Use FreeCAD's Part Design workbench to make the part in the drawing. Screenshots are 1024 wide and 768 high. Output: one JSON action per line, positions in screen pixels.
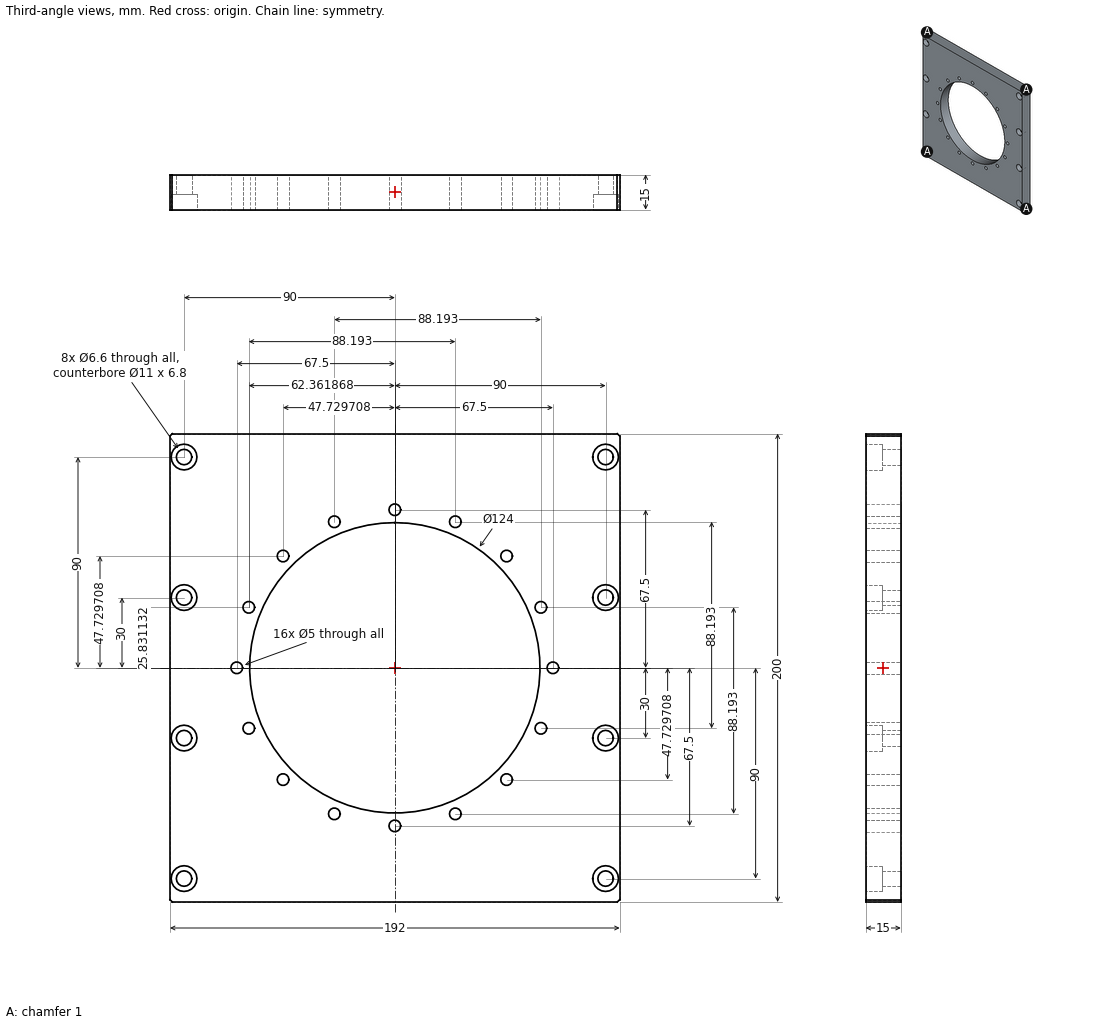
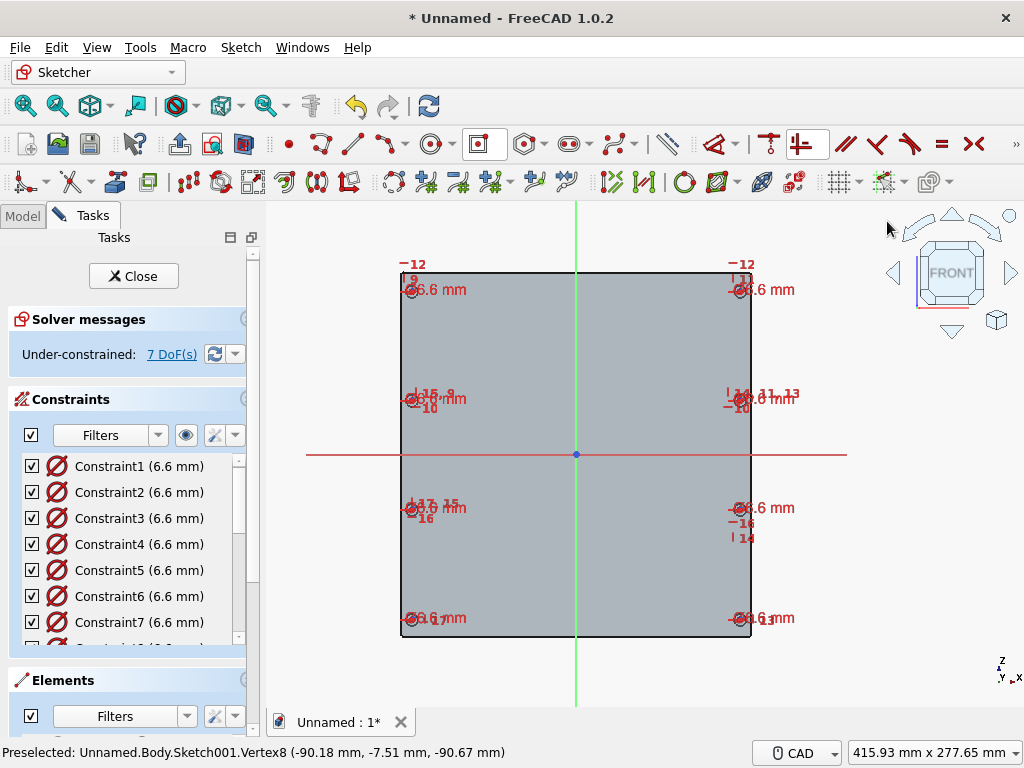
{"action": "left_click", "coordinate": [740, 620]}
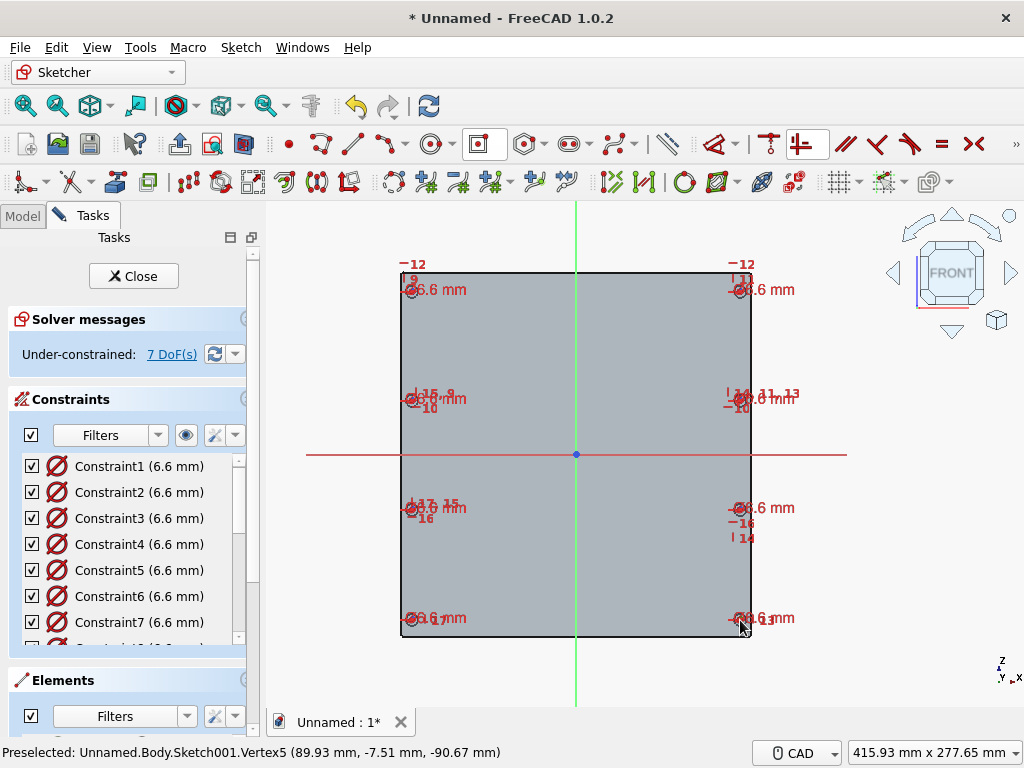
{"action": "left_click", "coordinate": [412, 620]}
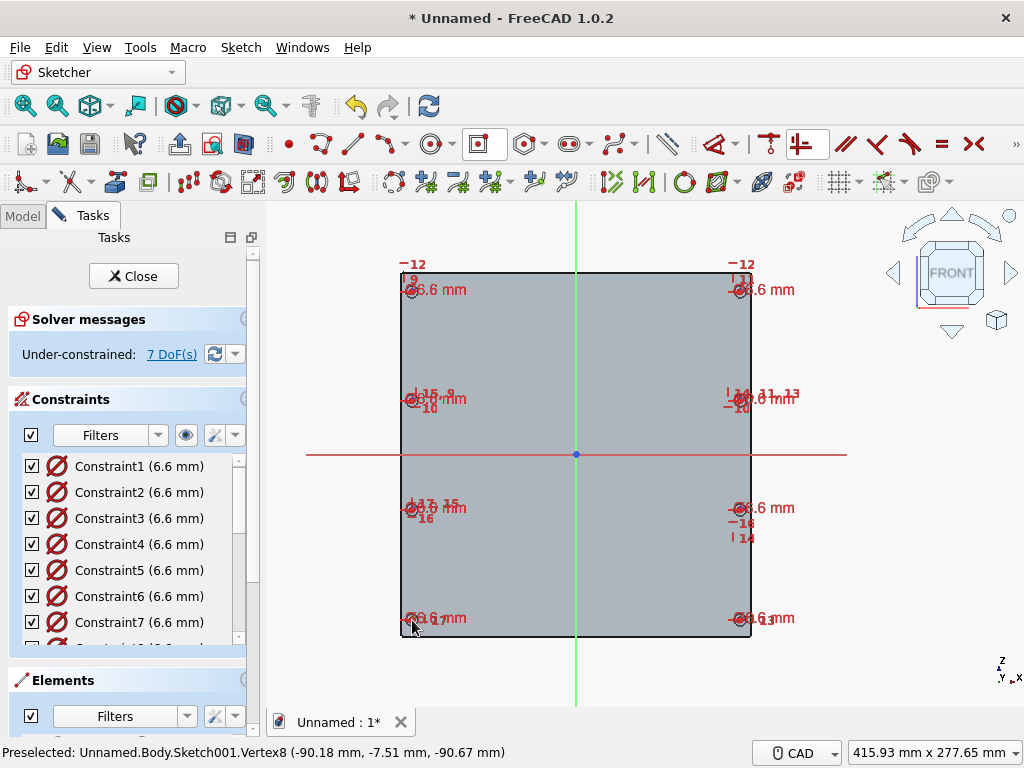
{"action": "key", "text": "h"}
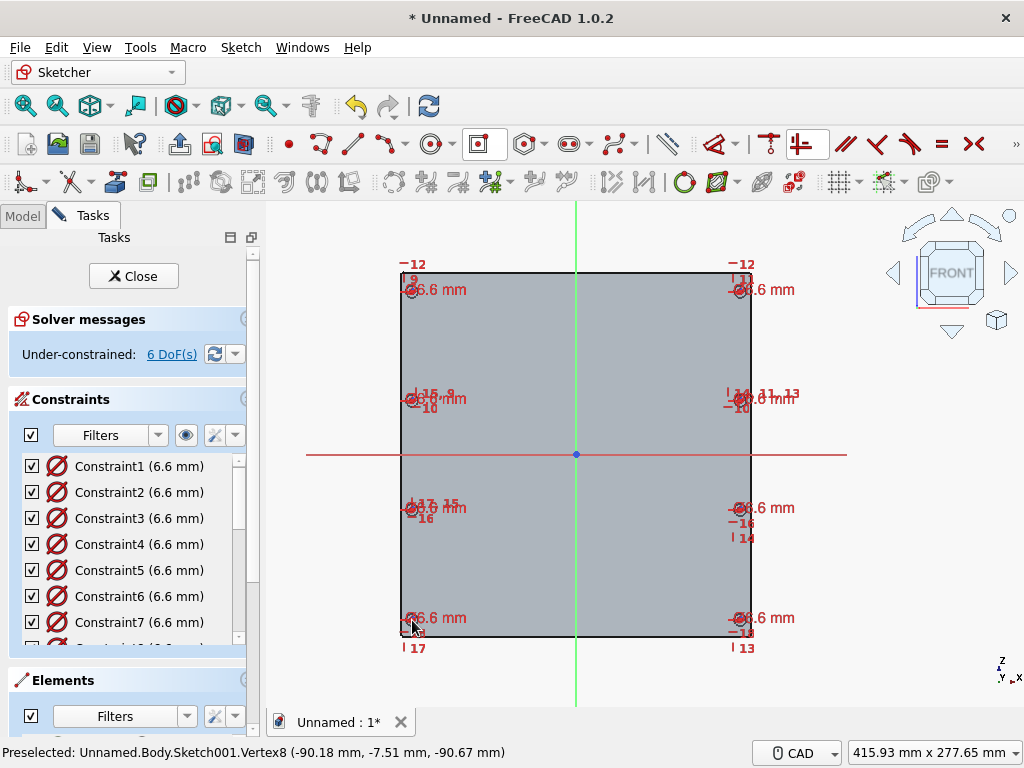
{"action": "left_click", "coordinate": [714, 144]}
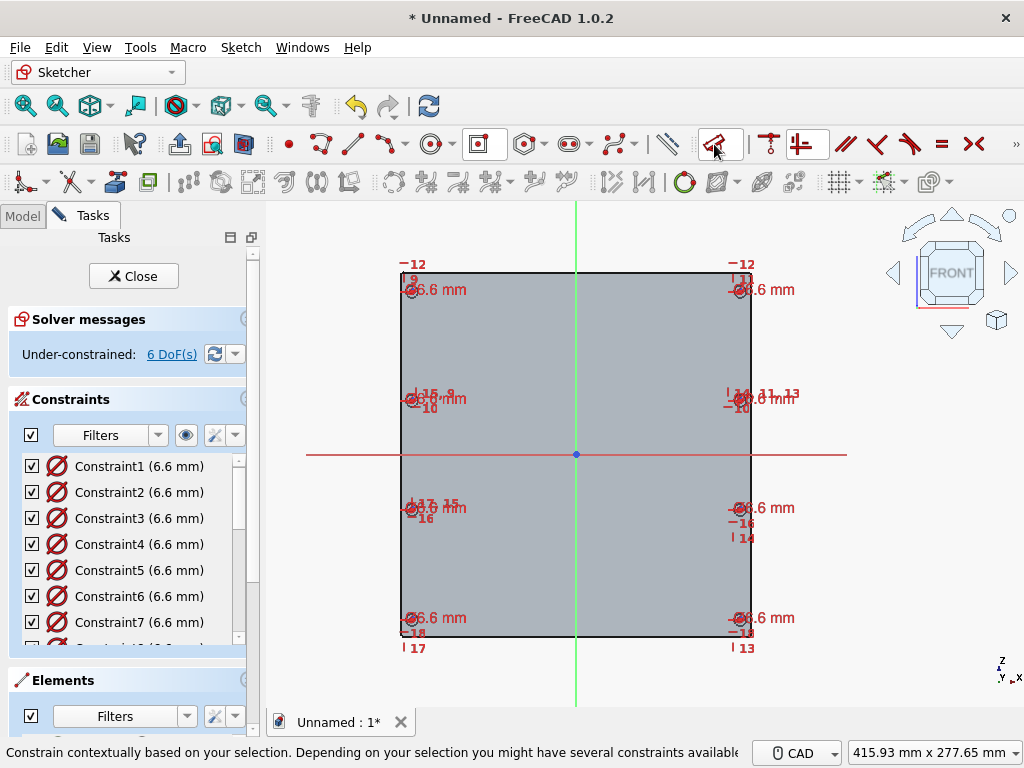
{"action": "left_click", "coordinate": [412, 292]}
{"action": "left_click", "coordinate": [494, 258]}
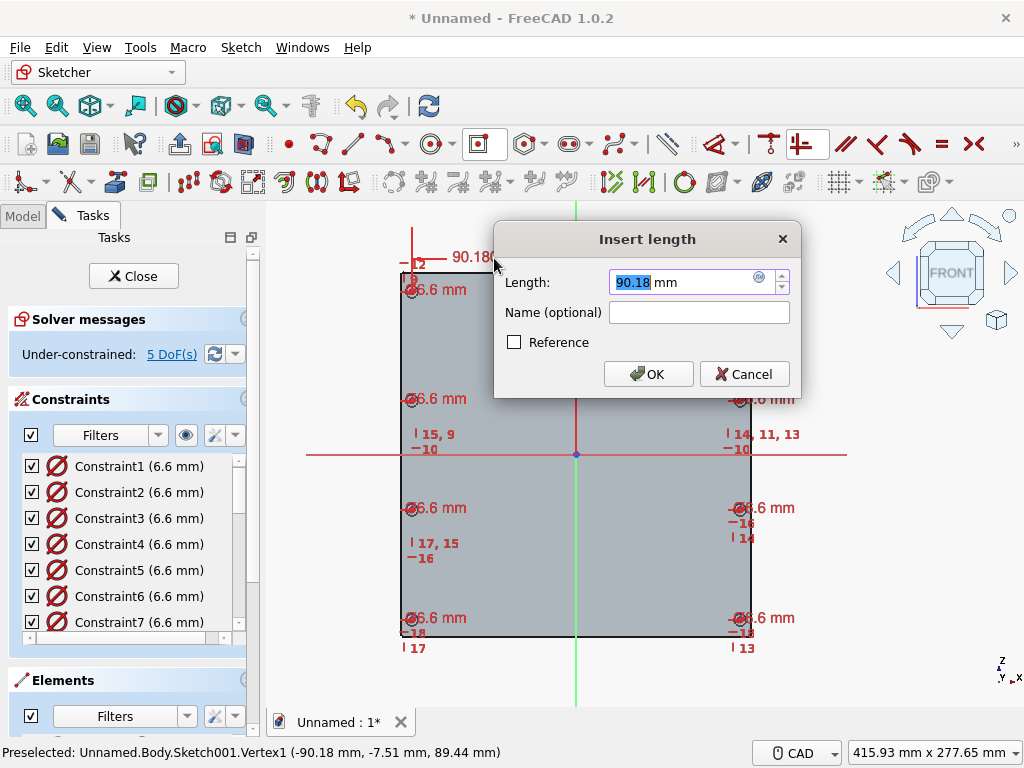
{"action": "type", "text": "90"}
{"action": "key", "text": "Return"}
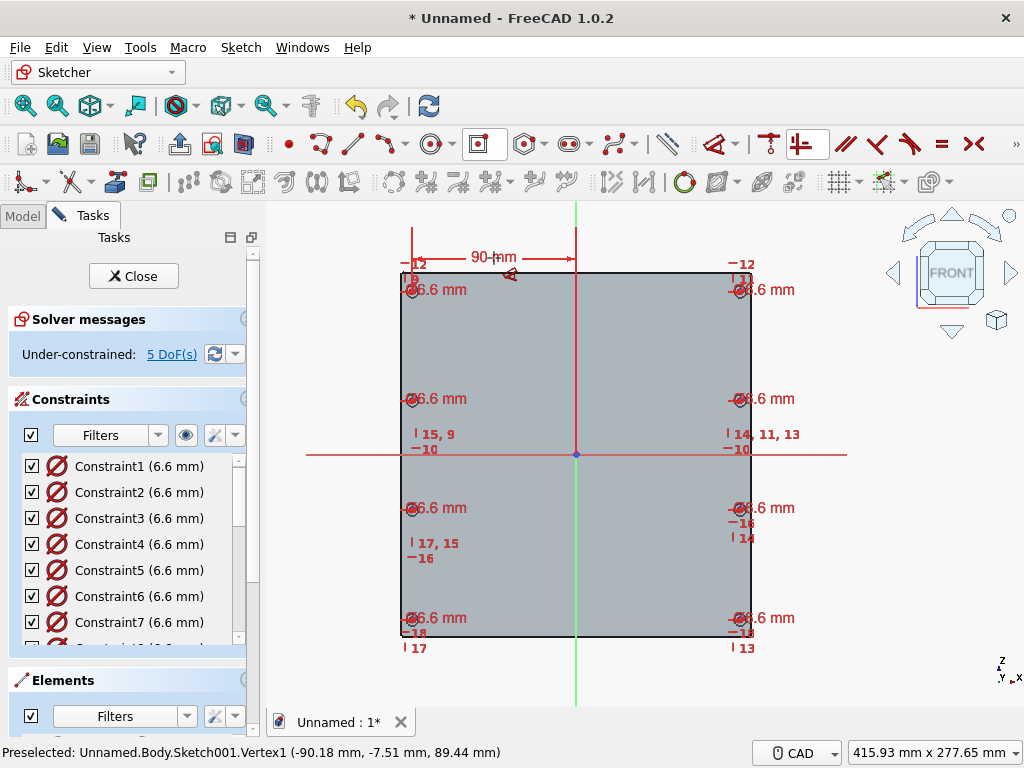
{"action": "left_click", "coordinate": [412, 292]}
{"action": "left_click", "coordinate": [378, 373]}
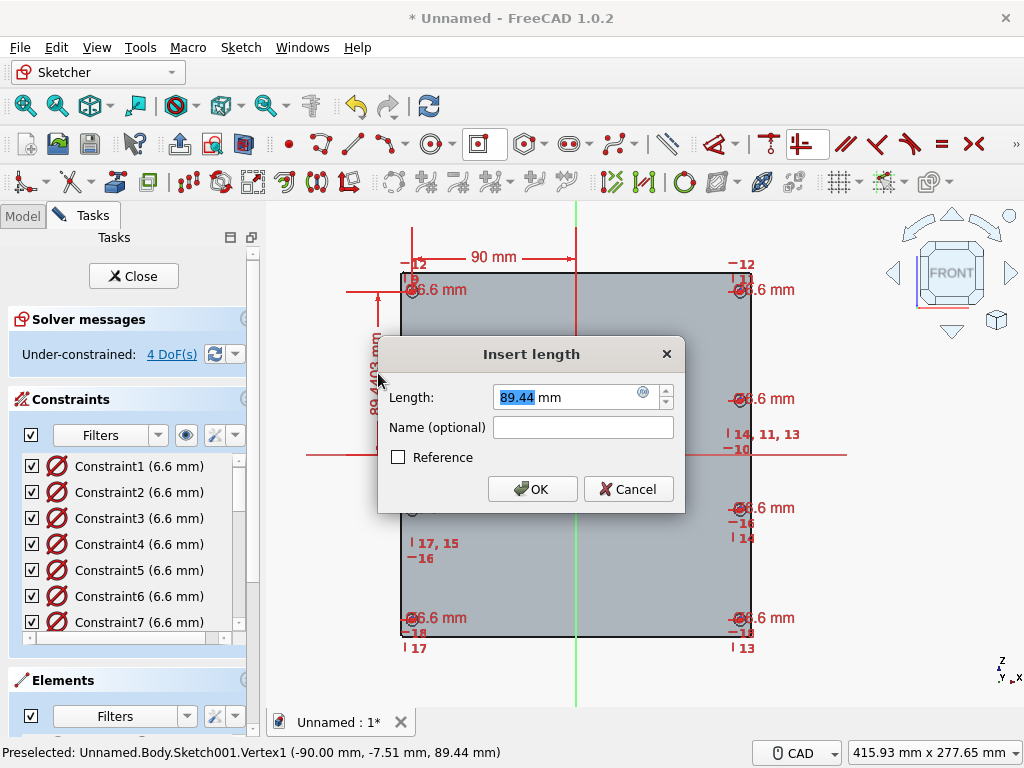
{"action": "type", "text": "90"}
{"action": "key", "text": "Return"}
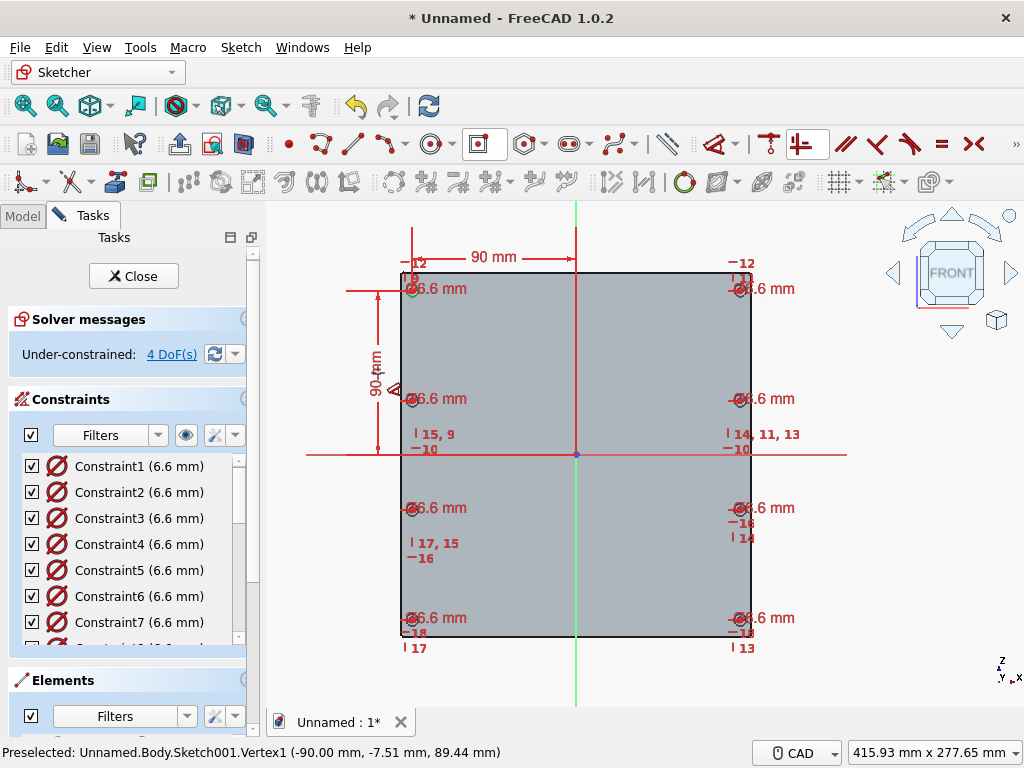
{"action": "left_click", "coordinate": [412, 401]}
{"action": "left_click", "coordinate": [378, 428]}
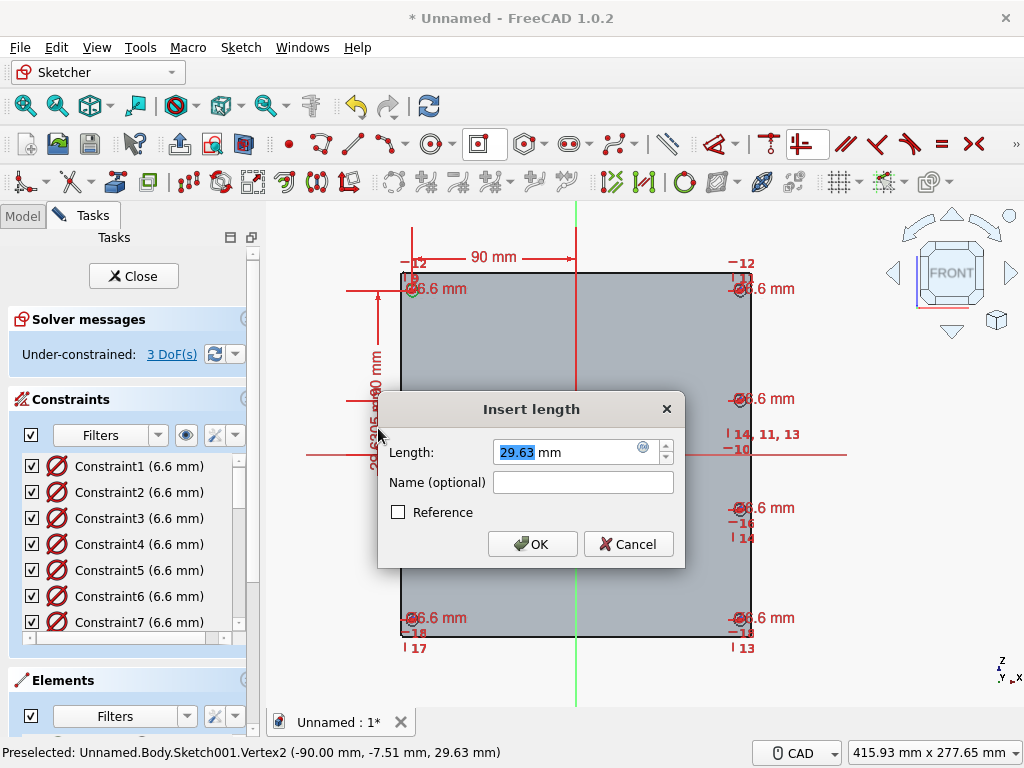
{"action": "type", "text": "30"}
{"action": "key", "text": "Return"}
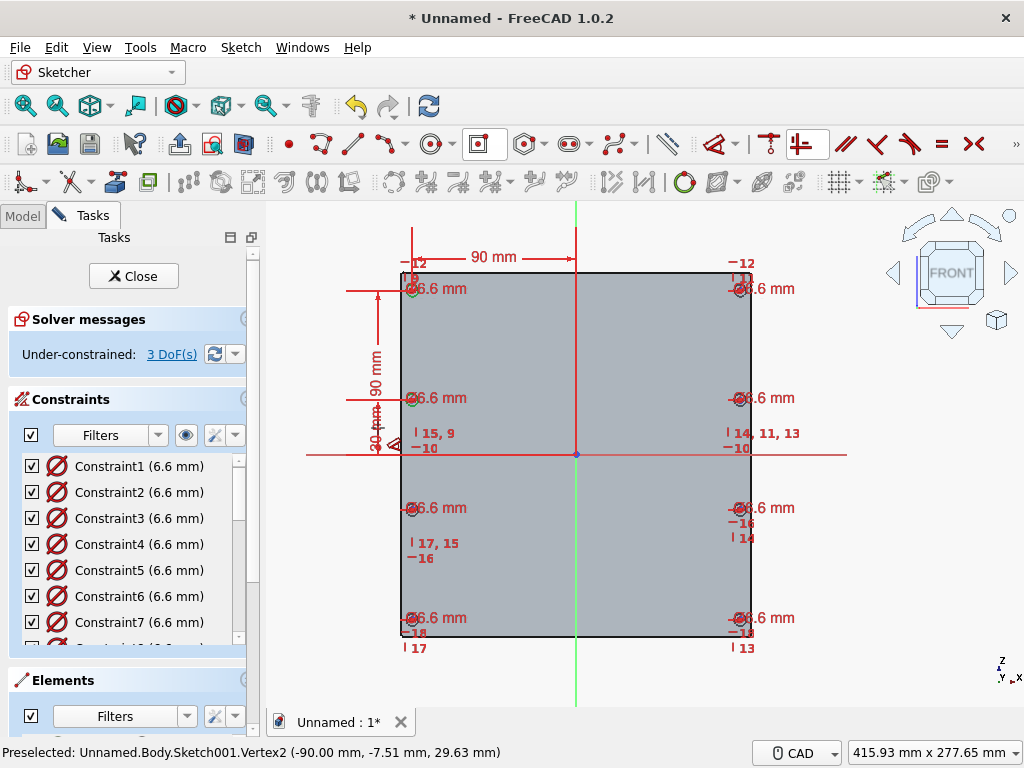
{"action": "left_click", "coordinate": [740, 400]}
{"action": "left_click", "coordinate": [658, 366]}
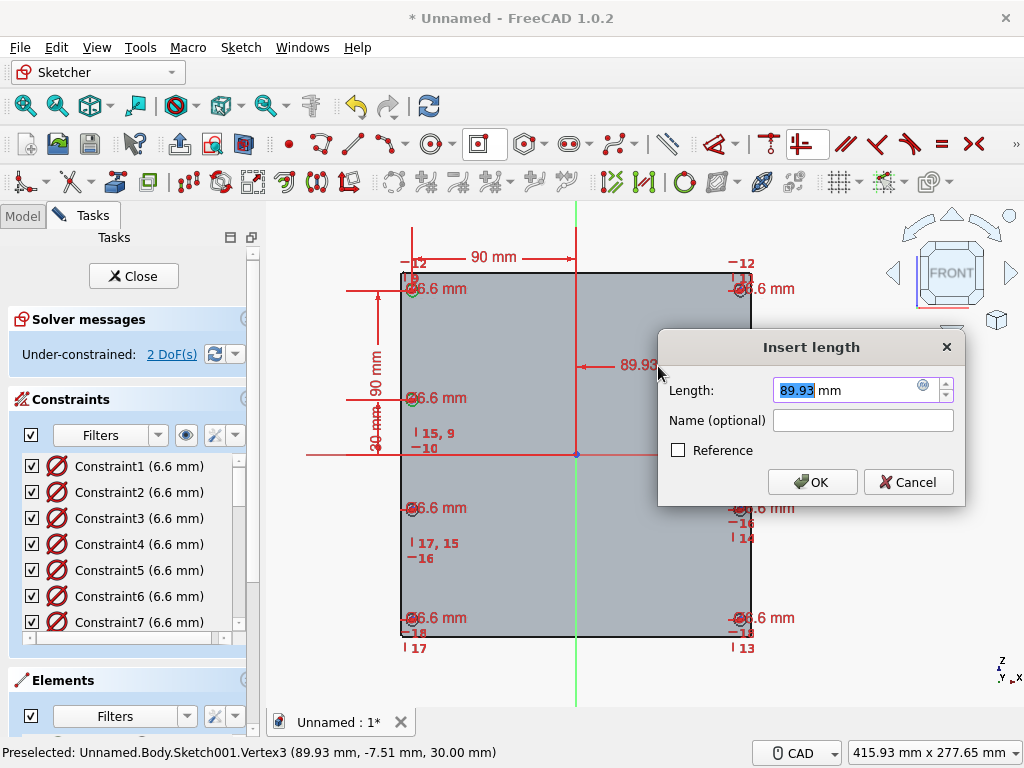
{"action": "type", "text": "90"}
{"action": "key", "text": "Return"}